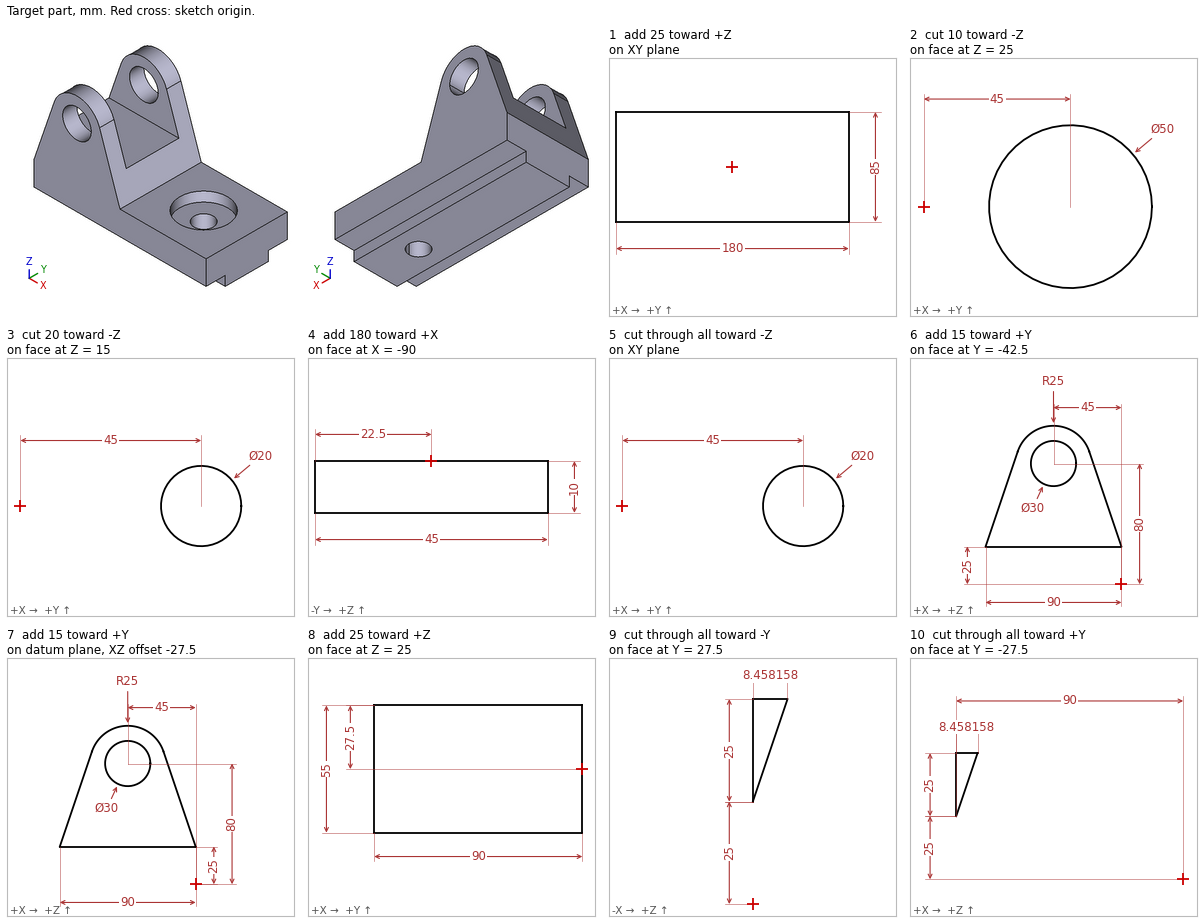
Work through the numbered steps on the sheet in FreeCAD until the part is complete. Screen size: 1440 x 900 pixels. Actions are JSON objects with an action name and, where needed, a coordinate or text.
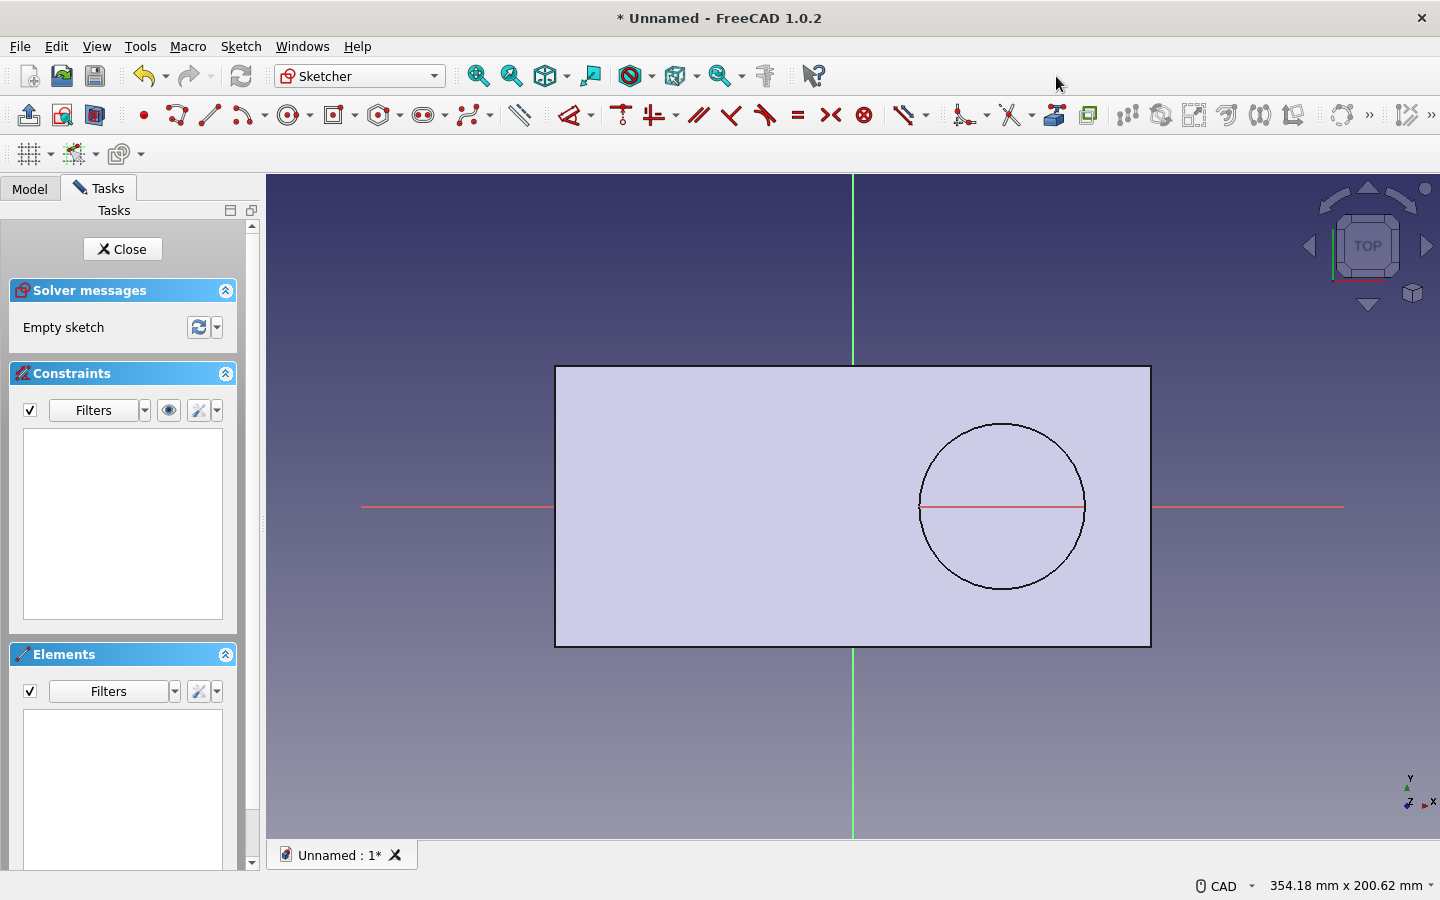
{"action": "scroll", "coordinate": [1045, 506], "scroll_direction": "up", "scroll_amount": 9}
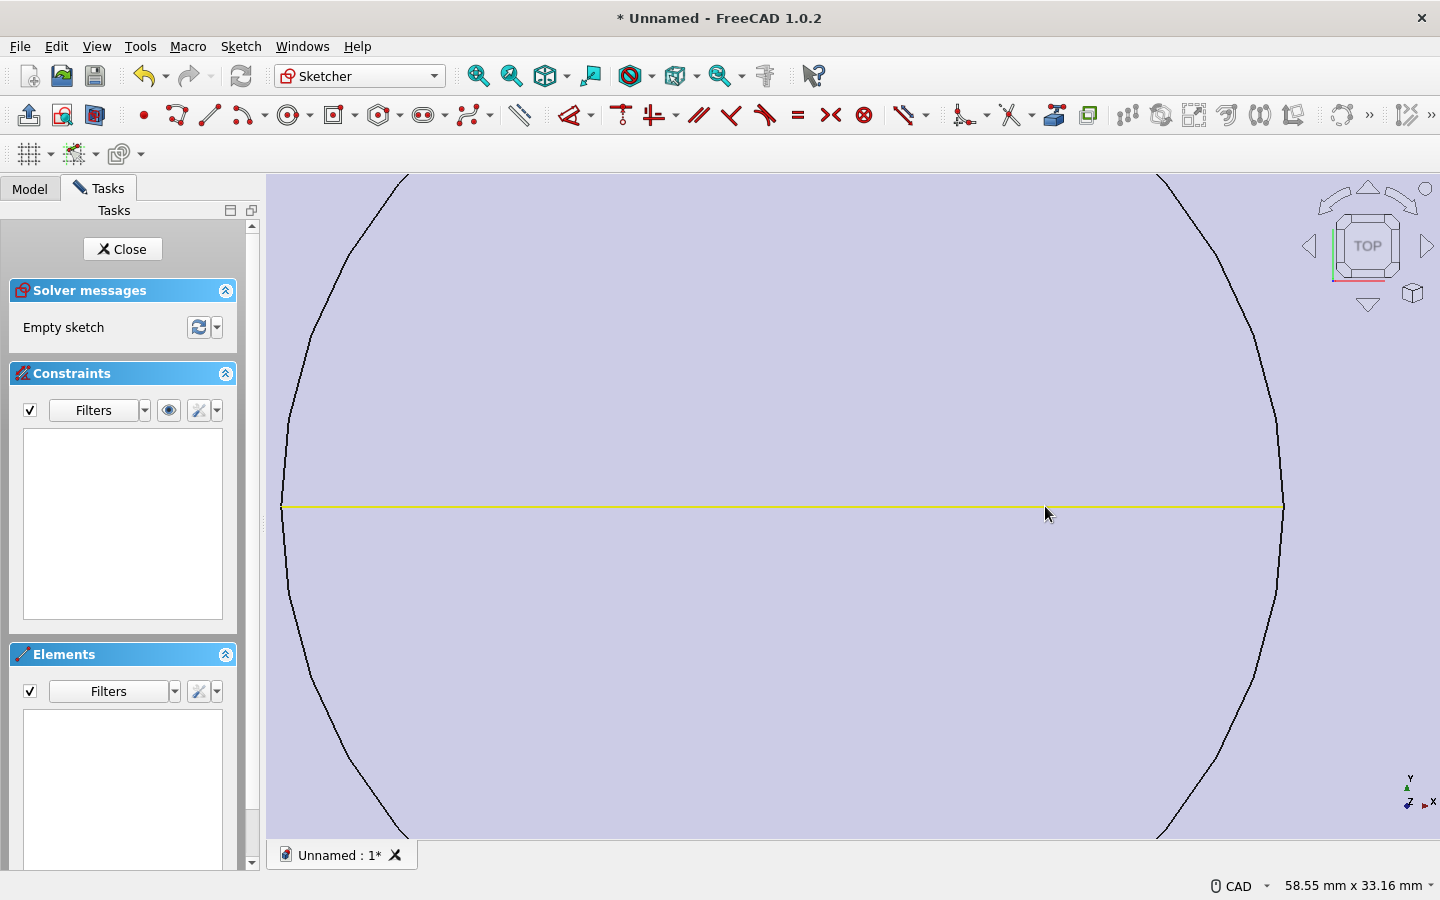
{"action": "left_click", "coordinate": [288, 116]}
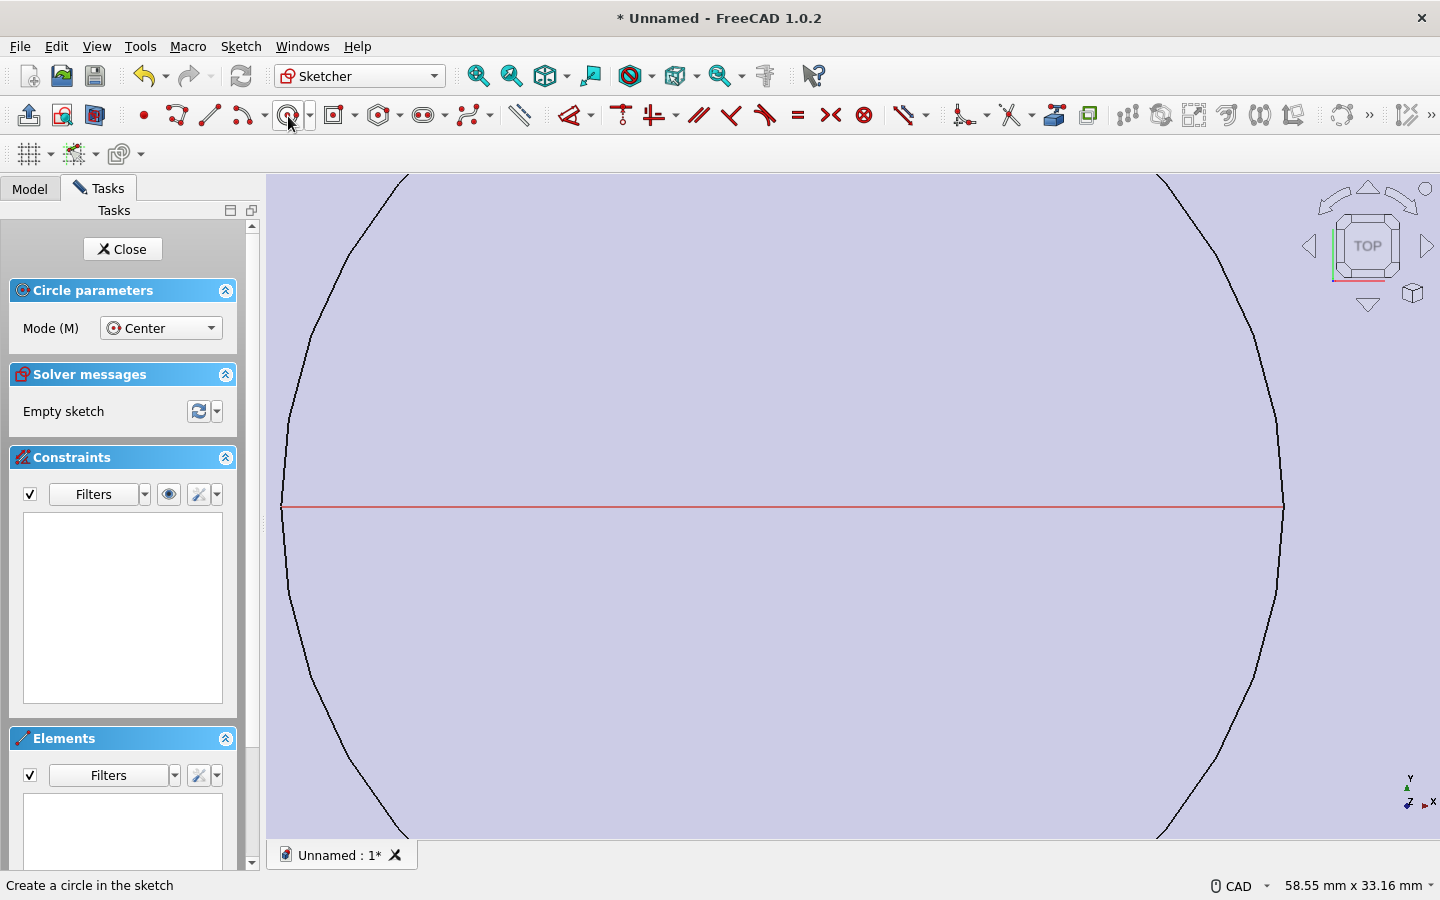
{"action": "left_click", "coordinate": [782, 506]}
{"action": "mouse_move", "coordinate": [924, 365]}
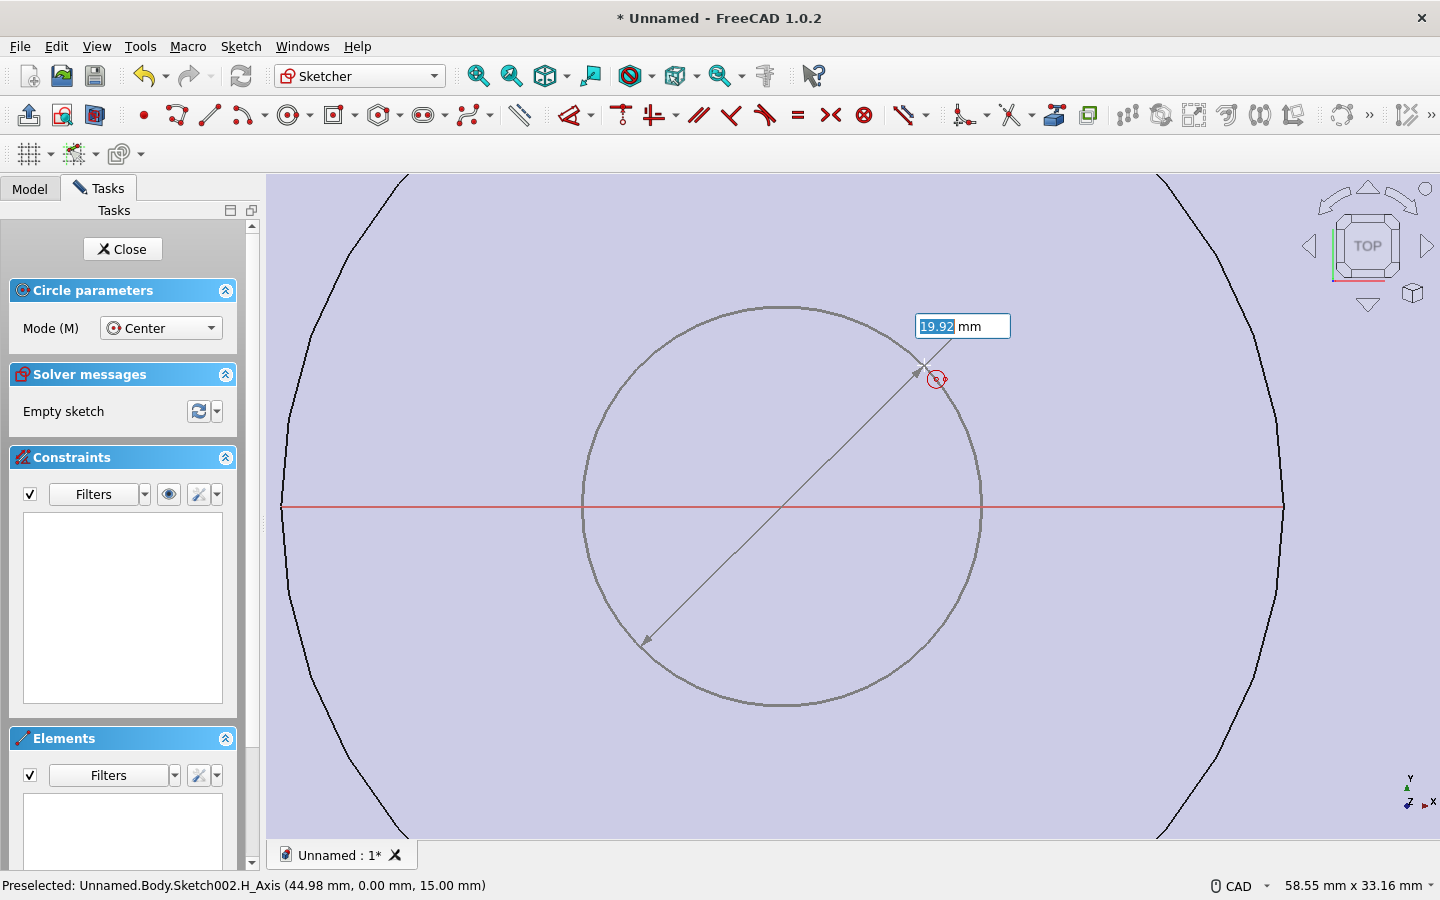
{"action": "type", "text": "20"}
{"action": "key", "text": "Return"}
{"action": "key", "text": "Escape"}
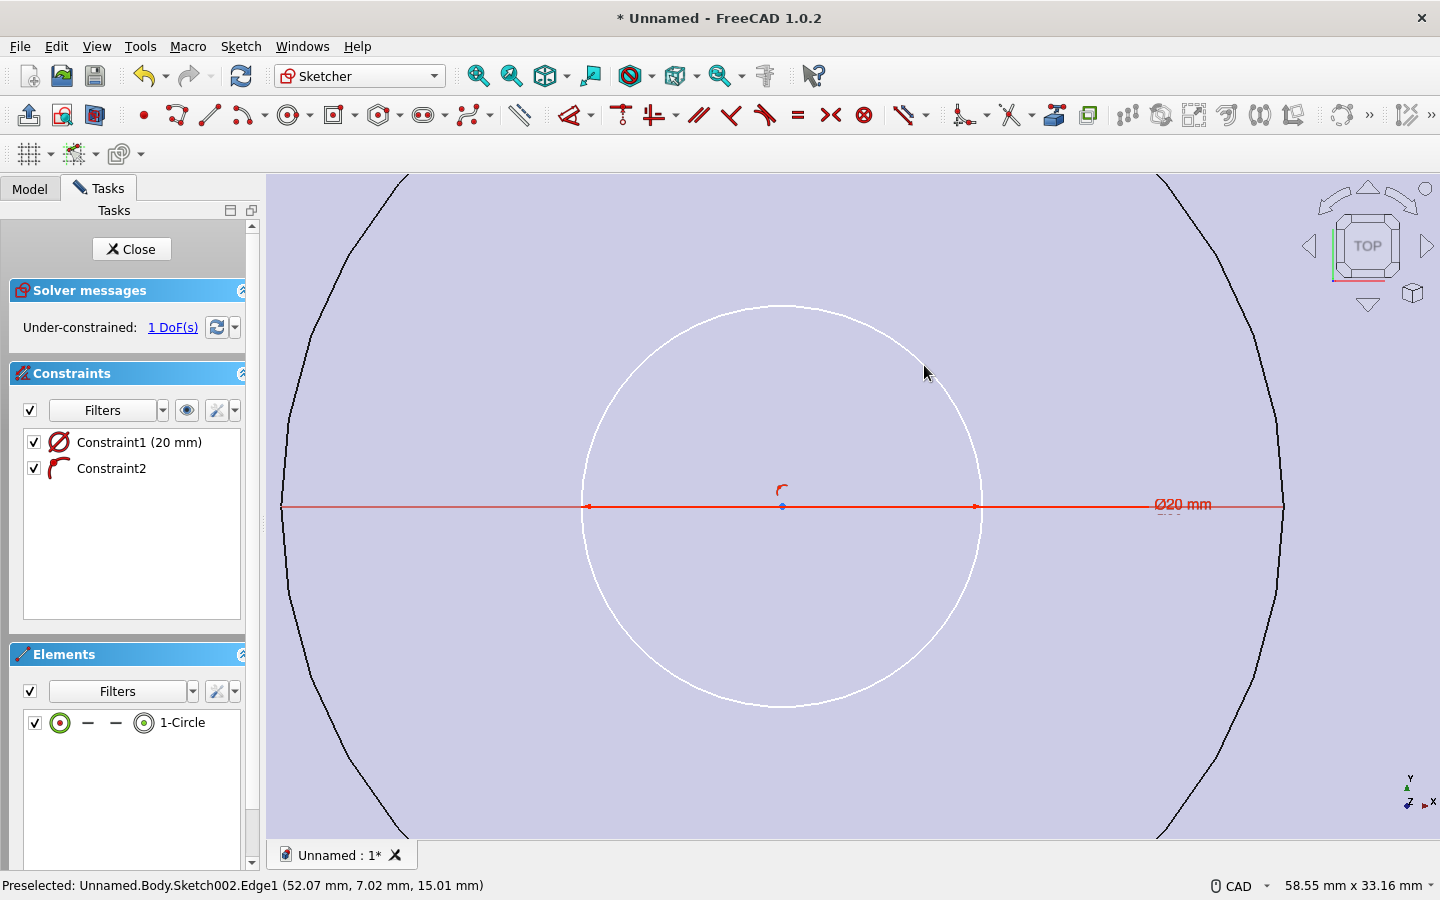
{"action": "left_click", "coordinate": [568, 116]}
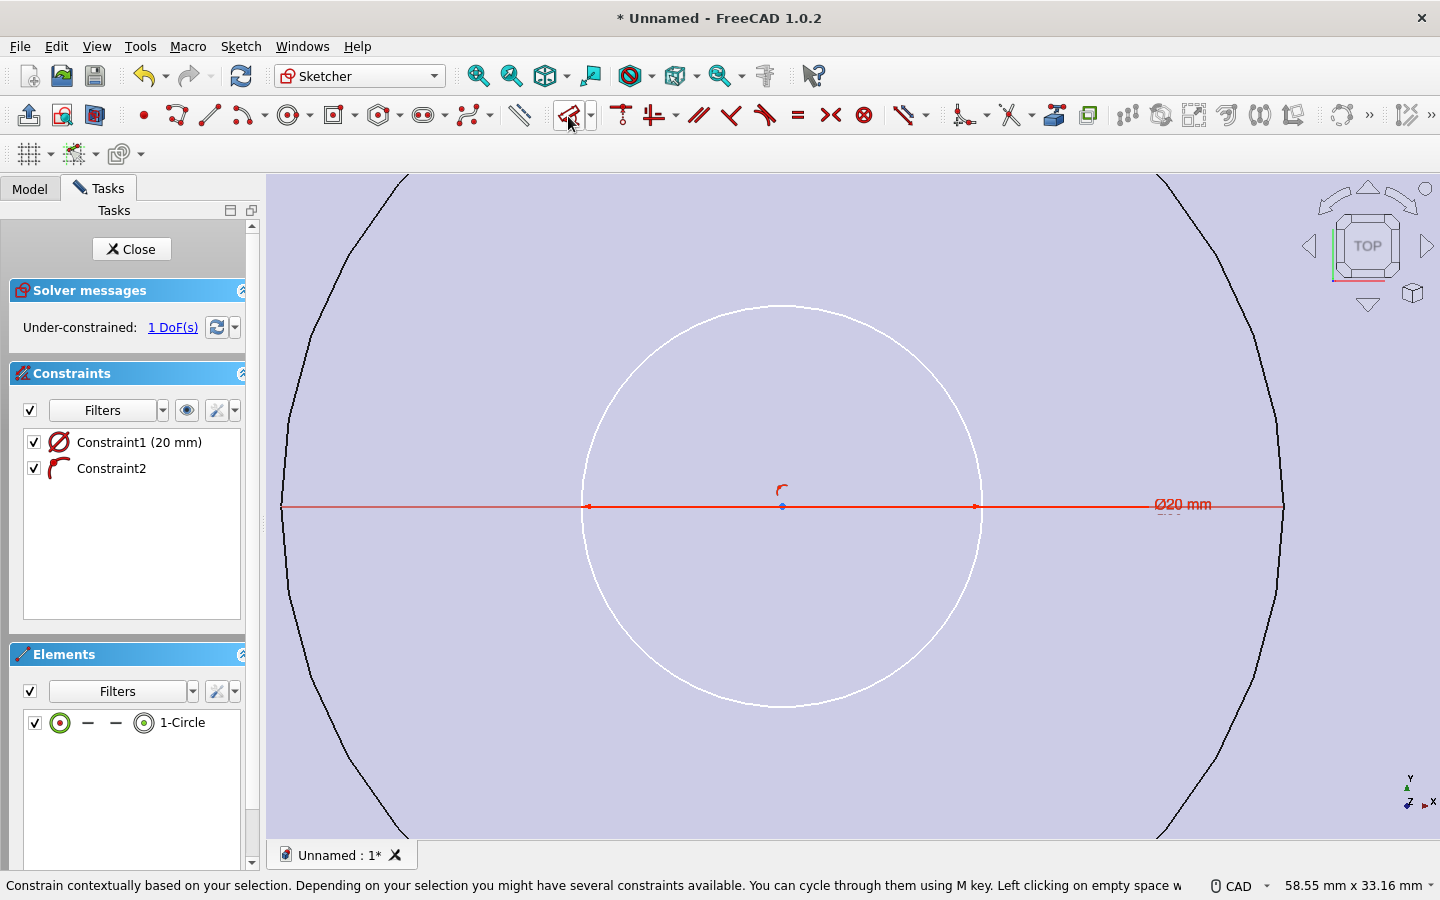
{"action": "left_click", "coordinate": [782, 506]}
{"action": "left_click", "coordinate": [538, 540]}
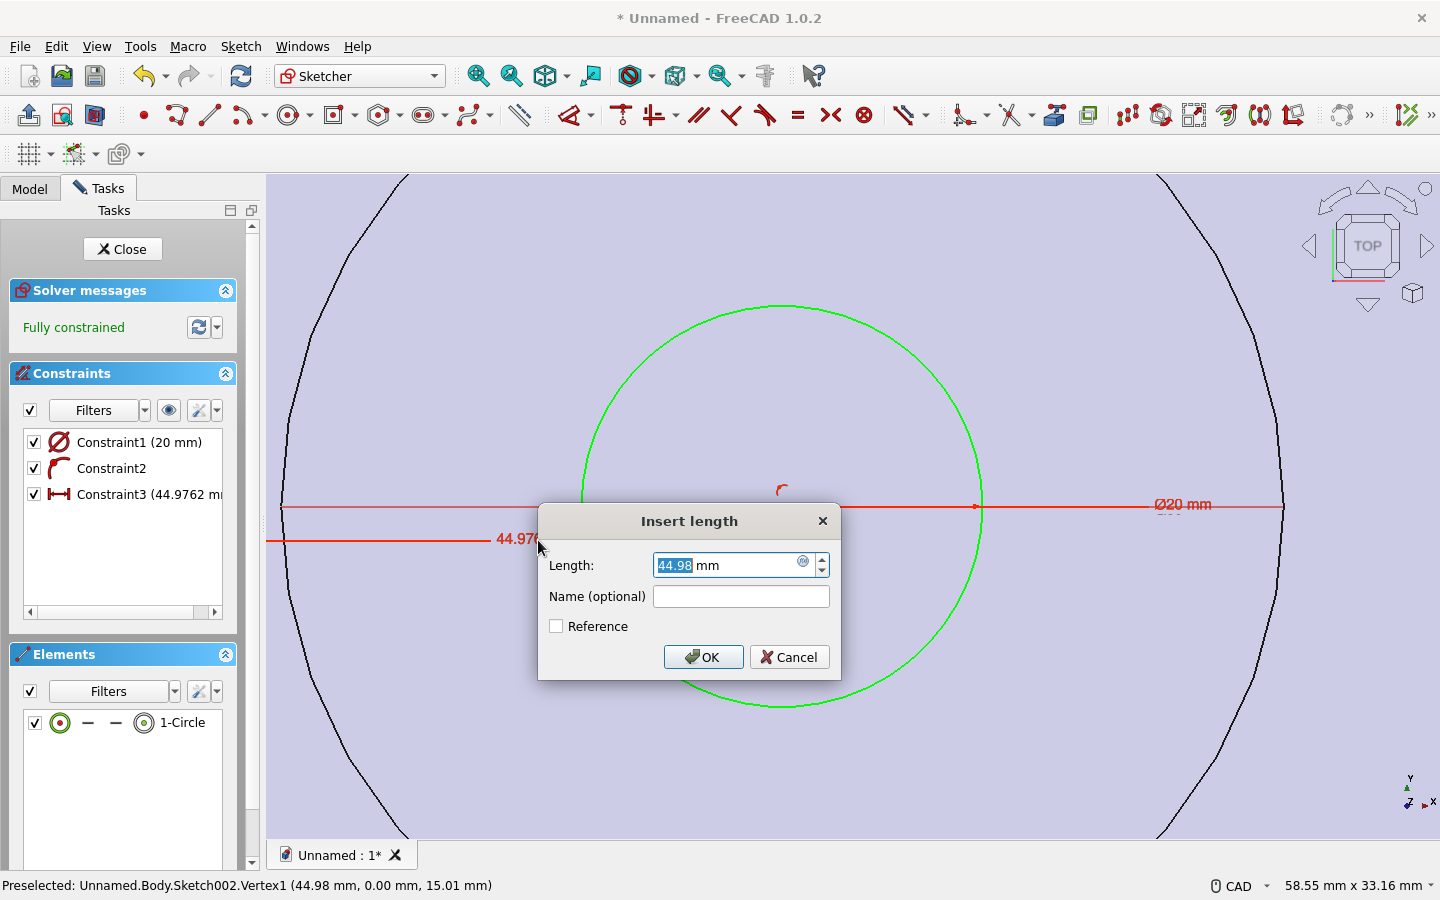
{"action": "type", "text": "45"}
{"action": "key", "text": "Return"}
{"action": "key", "text": "Escape"}